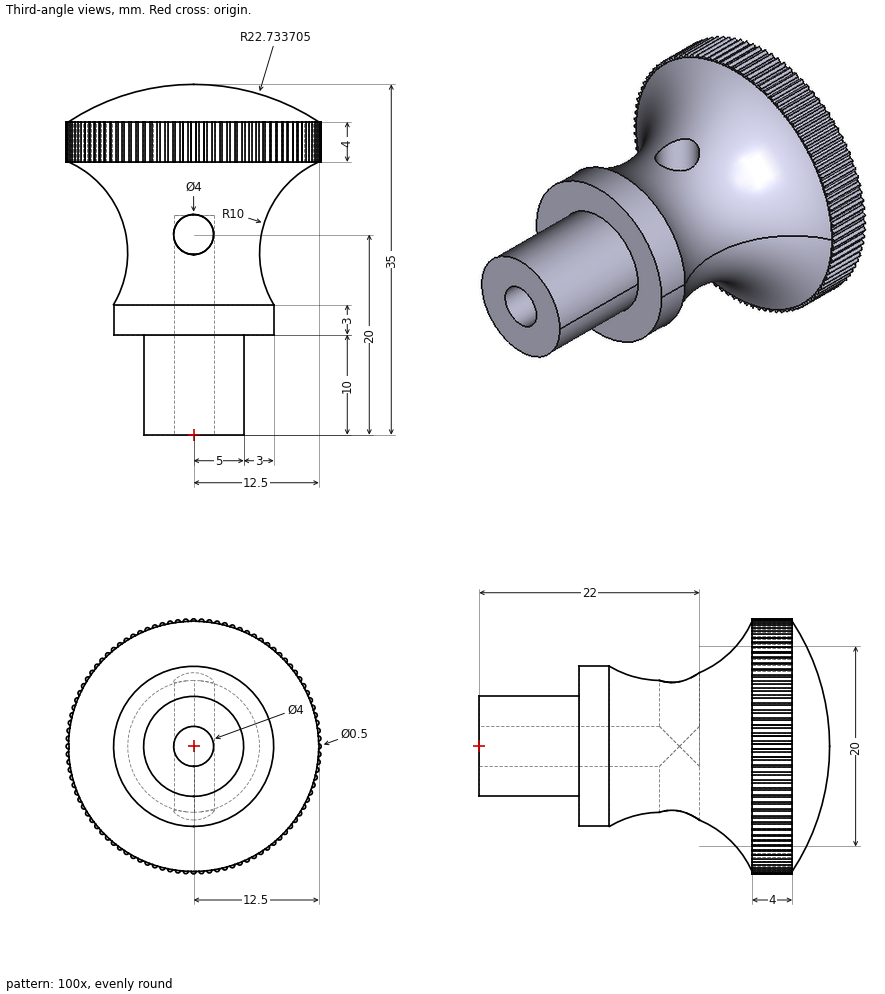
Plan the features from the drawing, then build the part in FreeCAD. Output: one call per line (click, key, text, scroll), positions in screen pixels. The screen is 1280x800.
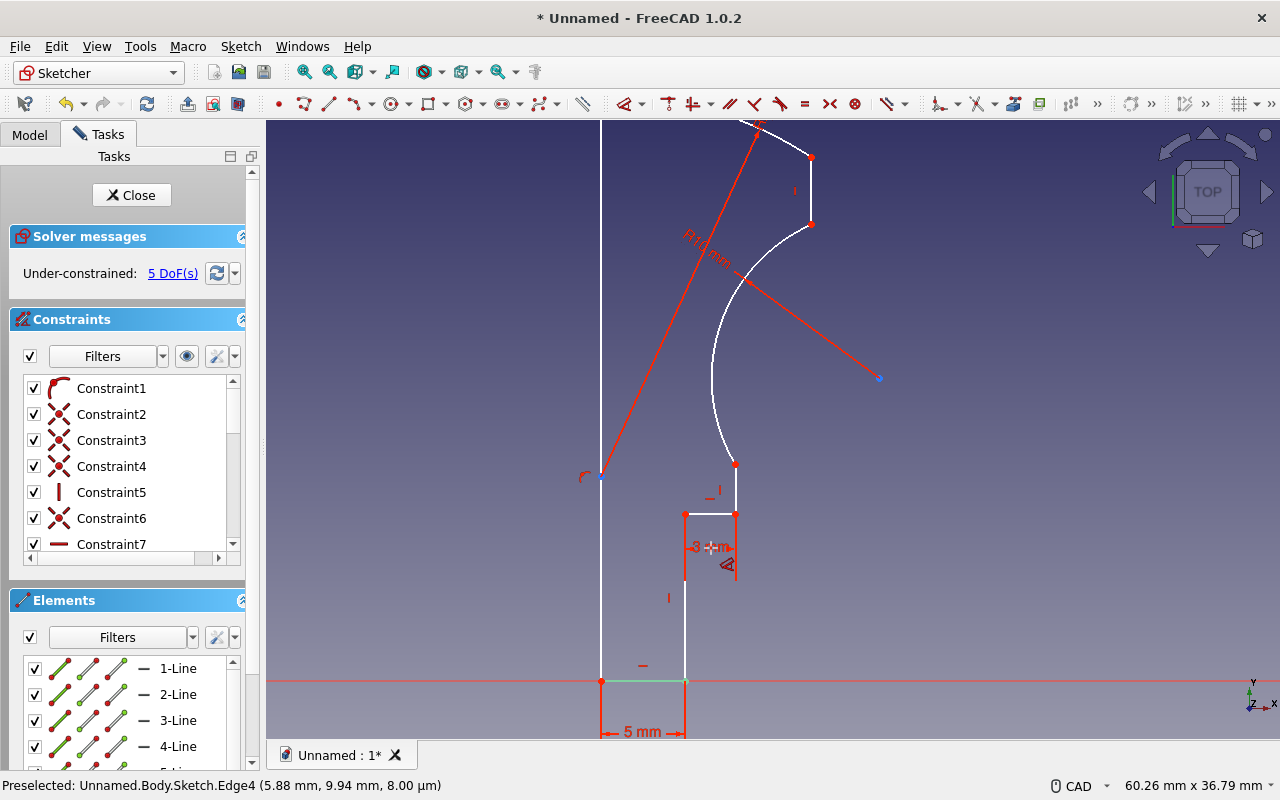
click(736, 499)
click(770, 490)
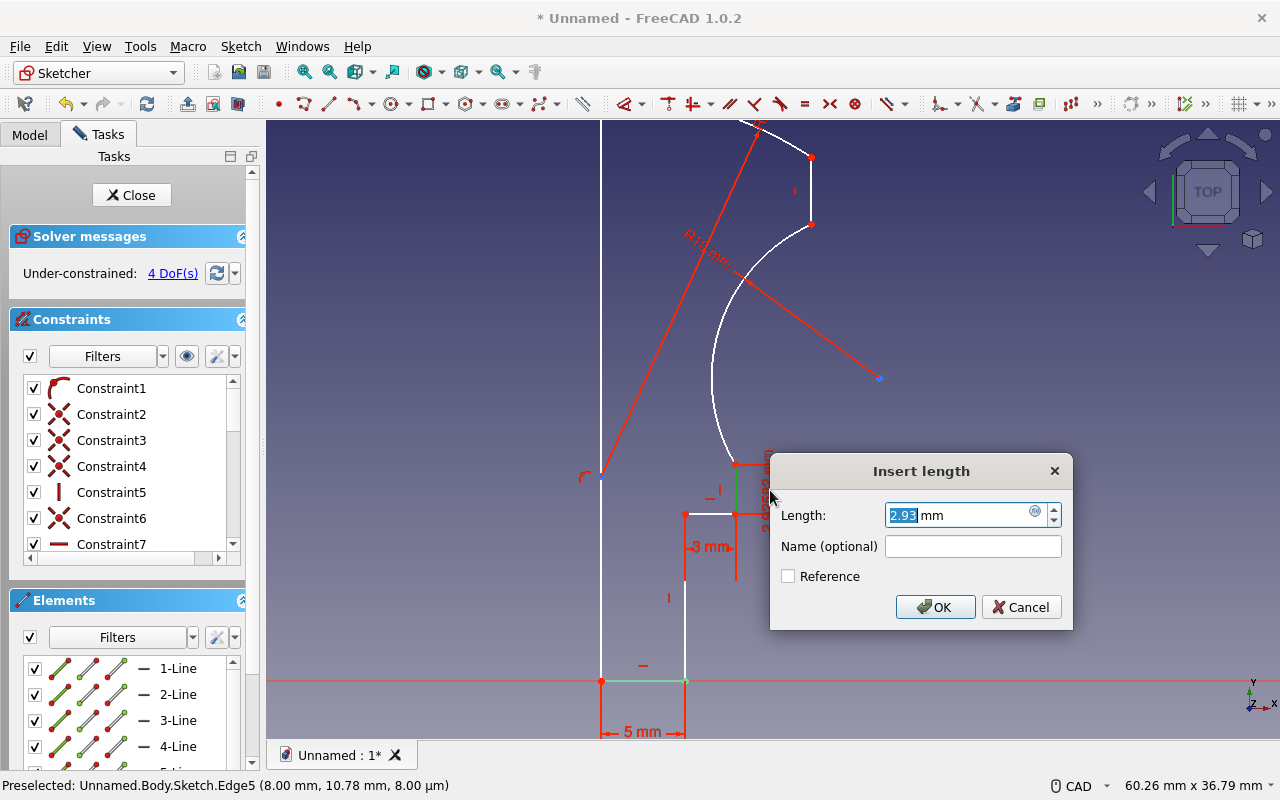
text(3)
key(Return)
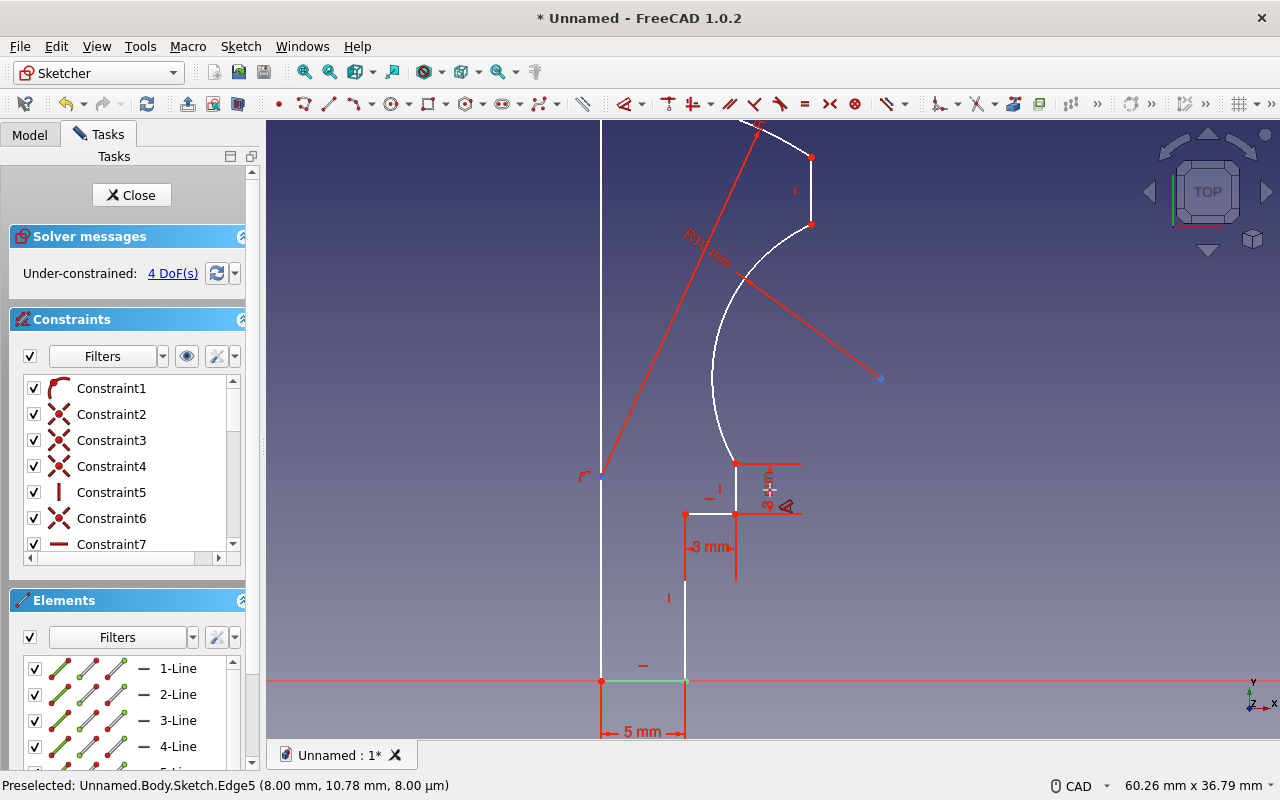
click(811, 204)
click(845, 191)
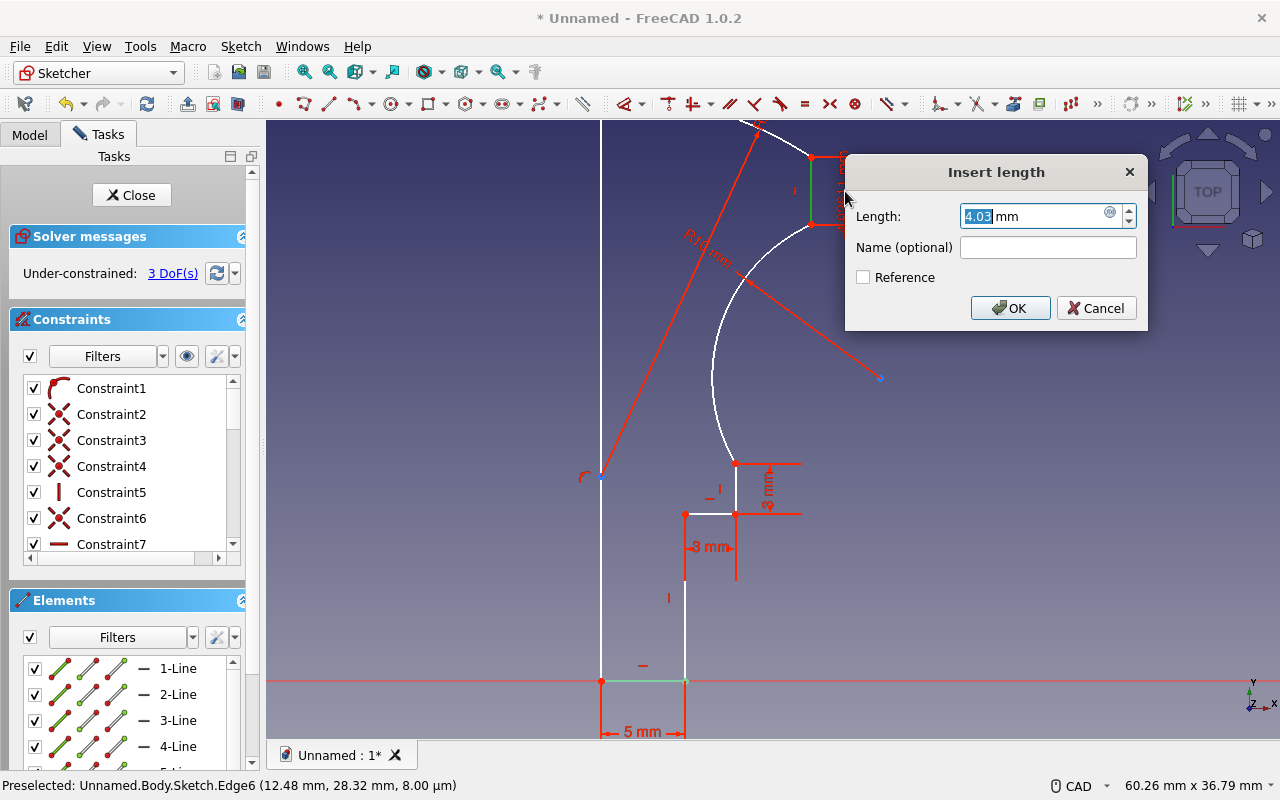
text(4)
key(Return)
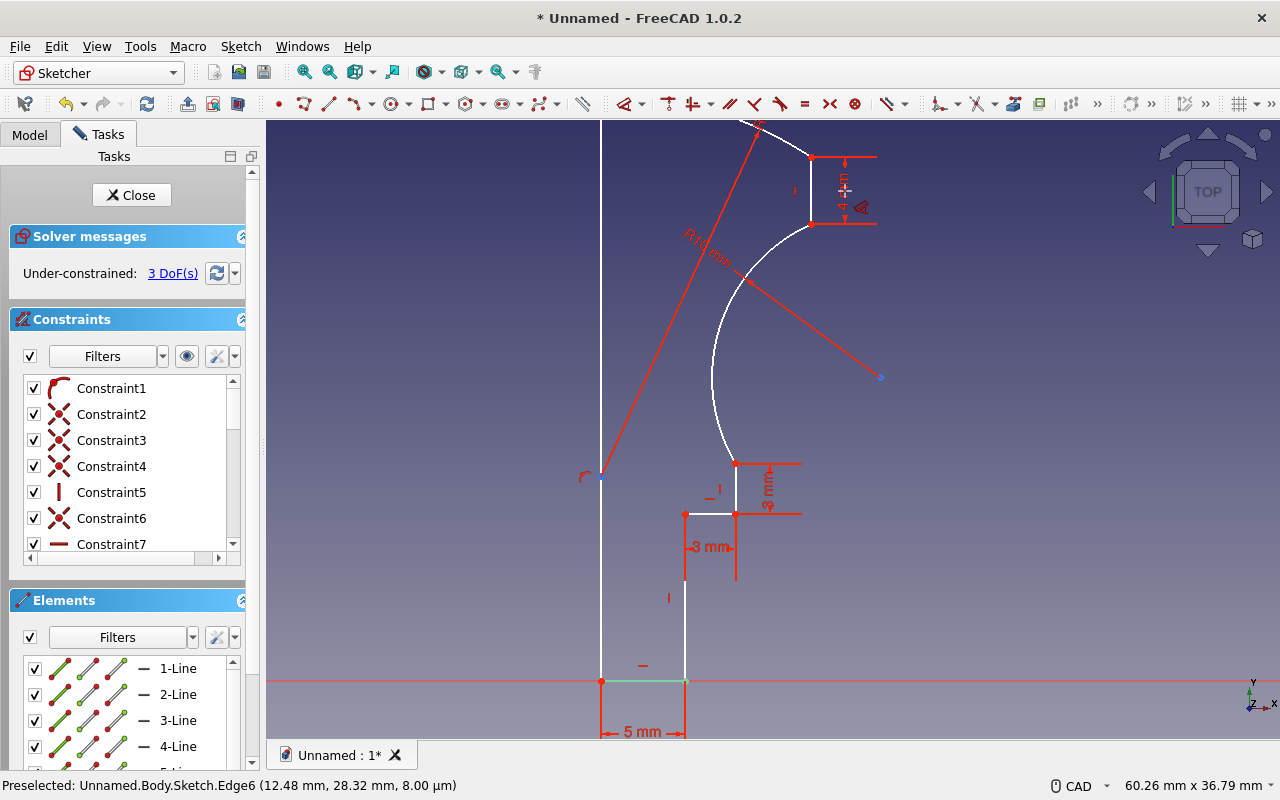
click(601, 270)
click(567, 415)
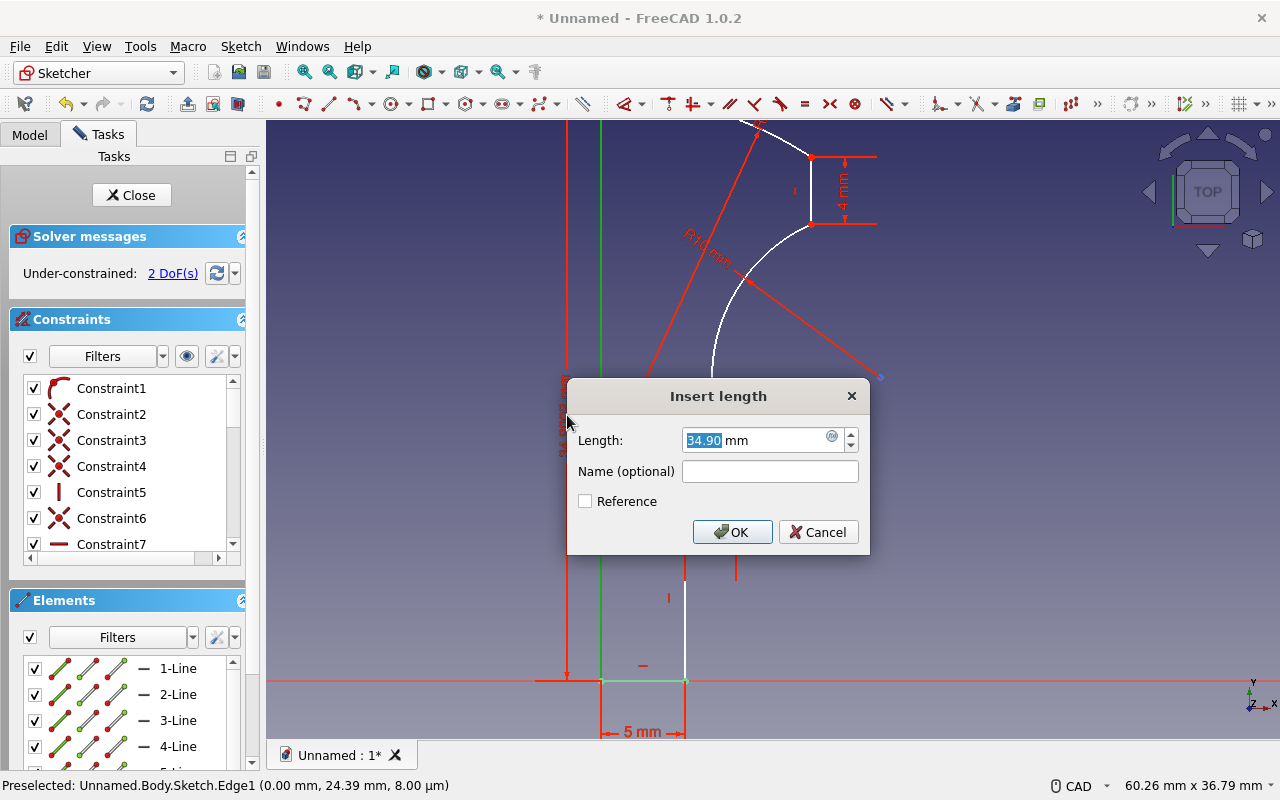
text(35)
key(Return)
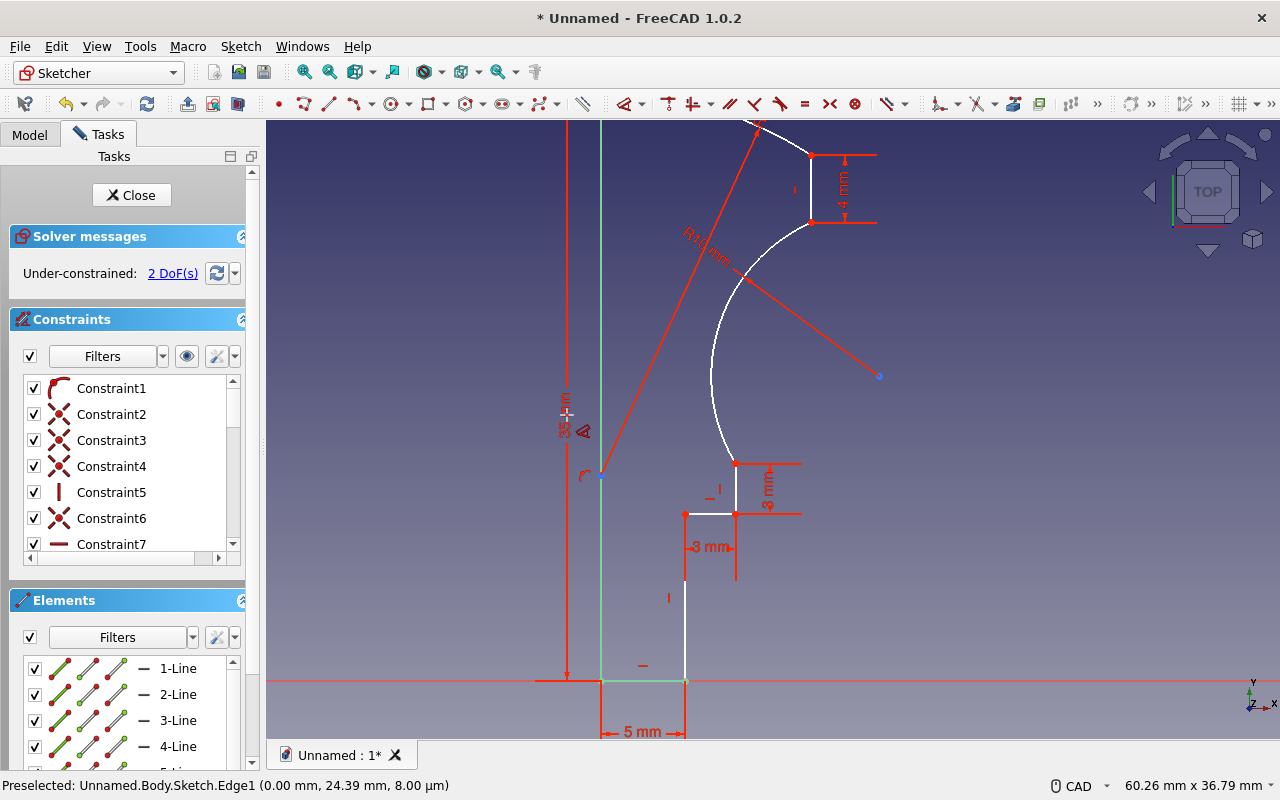
click(685, 631)
click(651, 598)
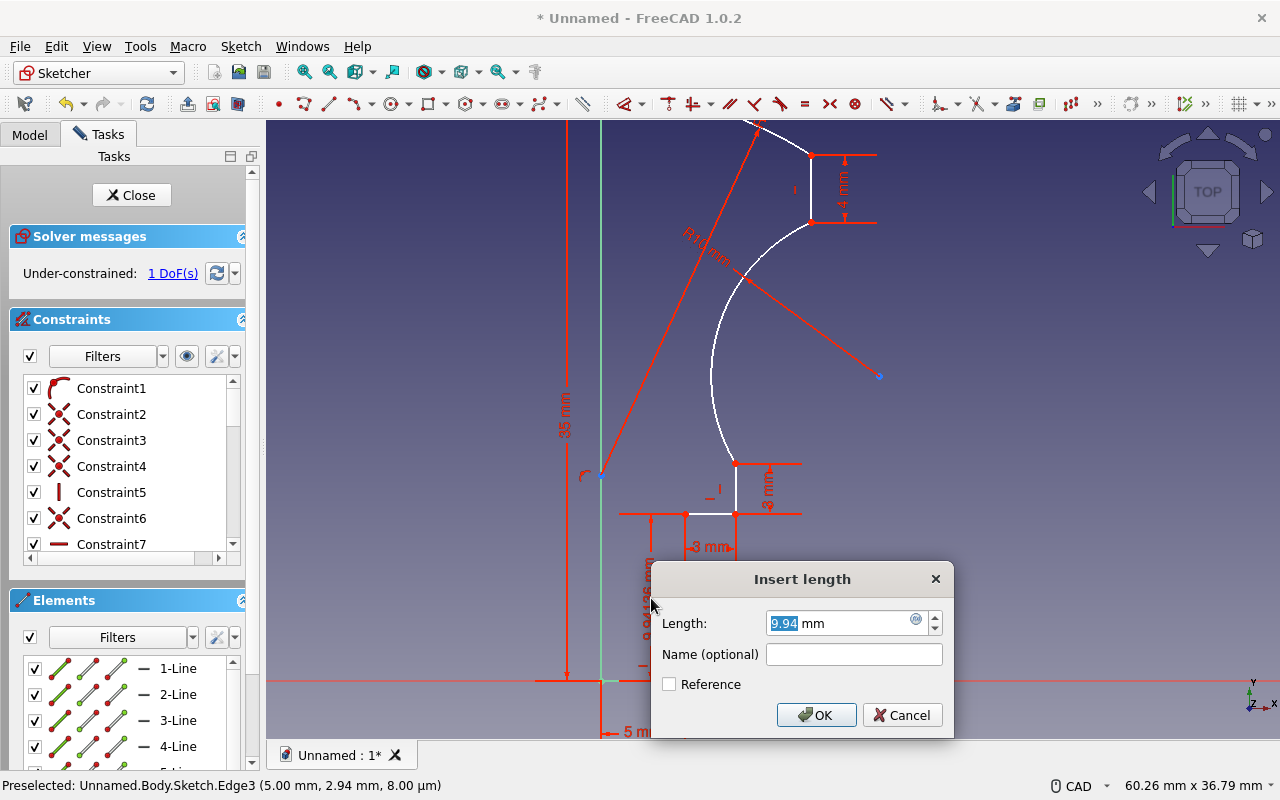
text(10)
key(Return)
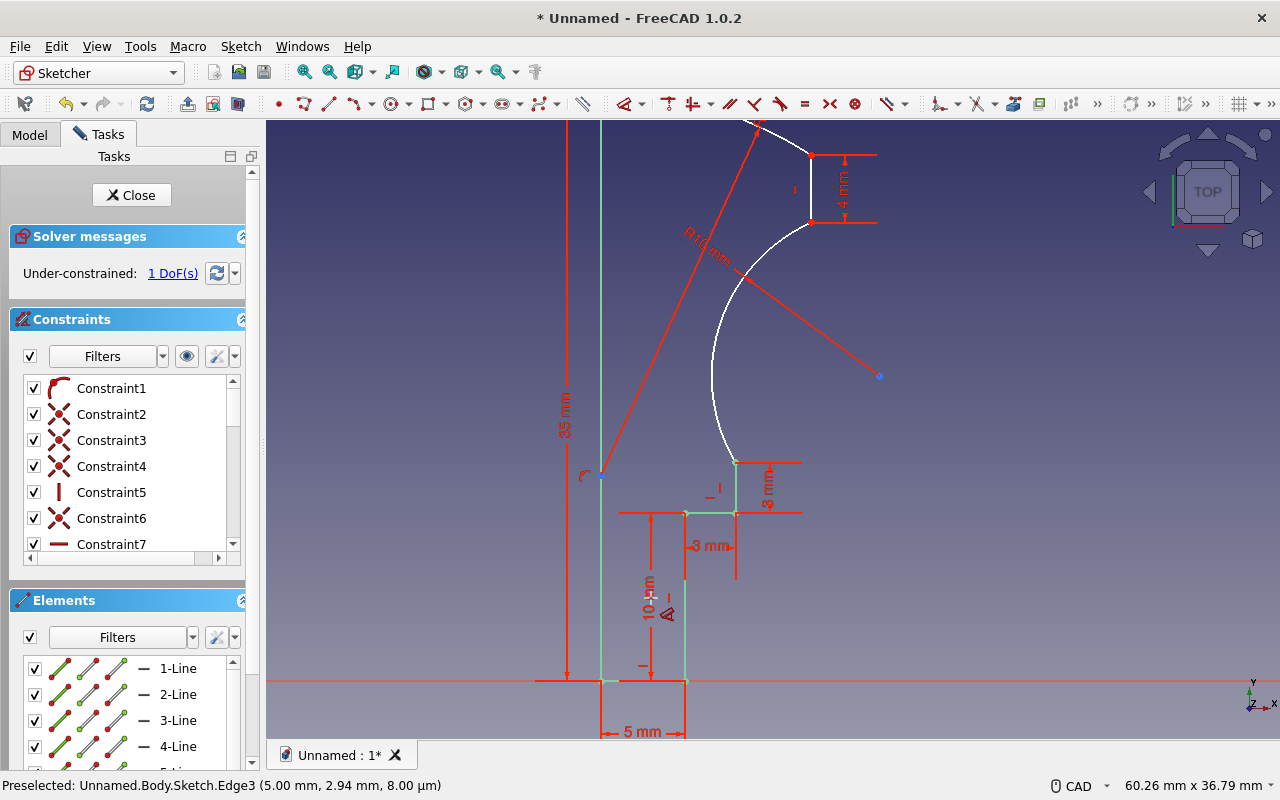
click(811, 223)
click(706, 189)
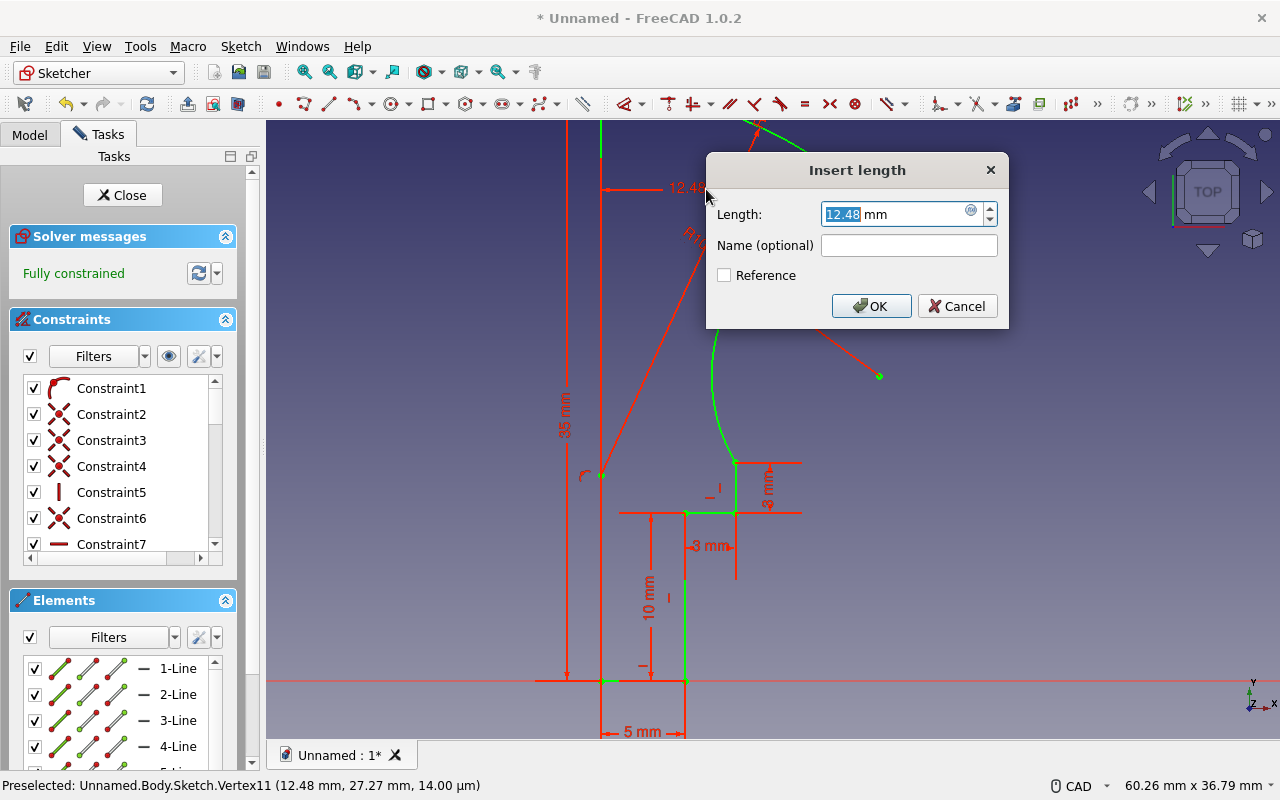
text(12.5)
key(Return)
key(Escape)